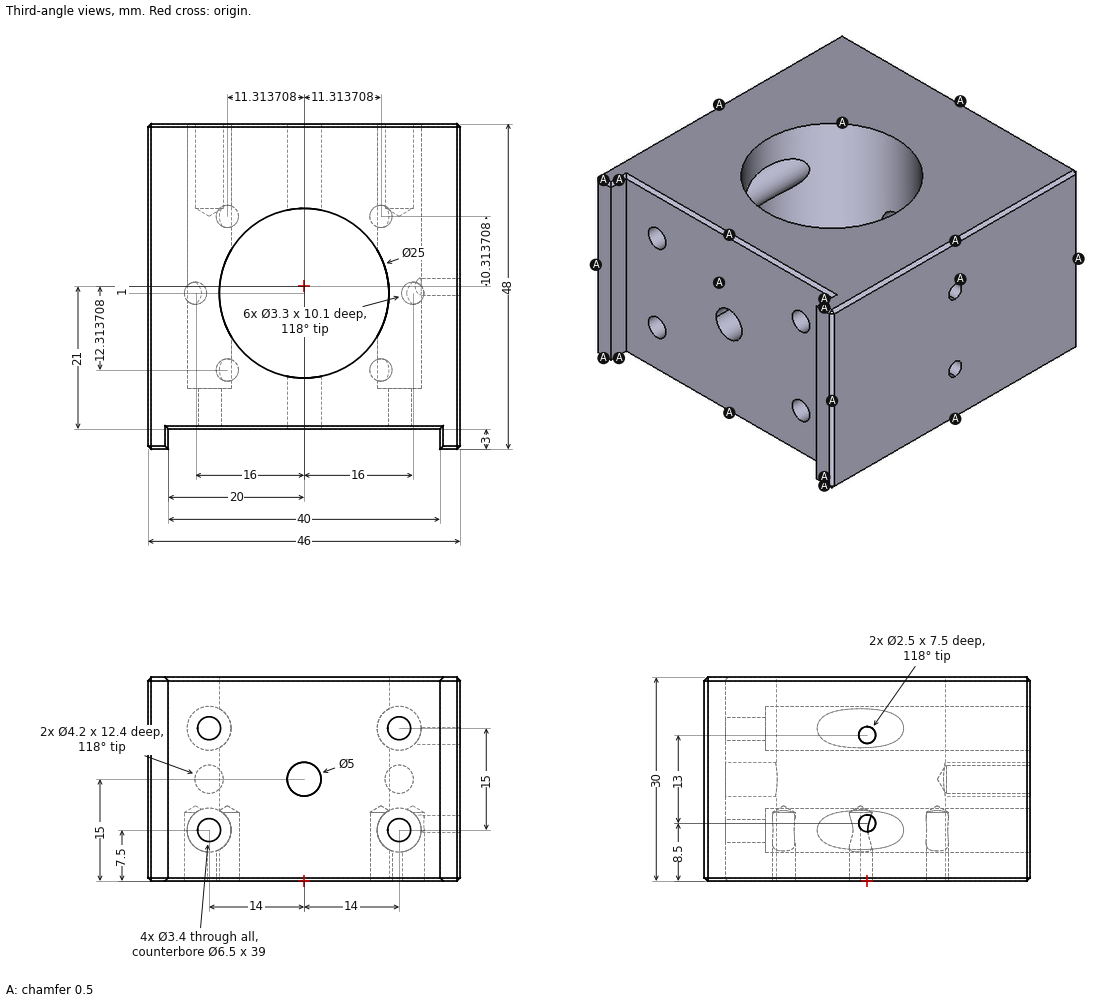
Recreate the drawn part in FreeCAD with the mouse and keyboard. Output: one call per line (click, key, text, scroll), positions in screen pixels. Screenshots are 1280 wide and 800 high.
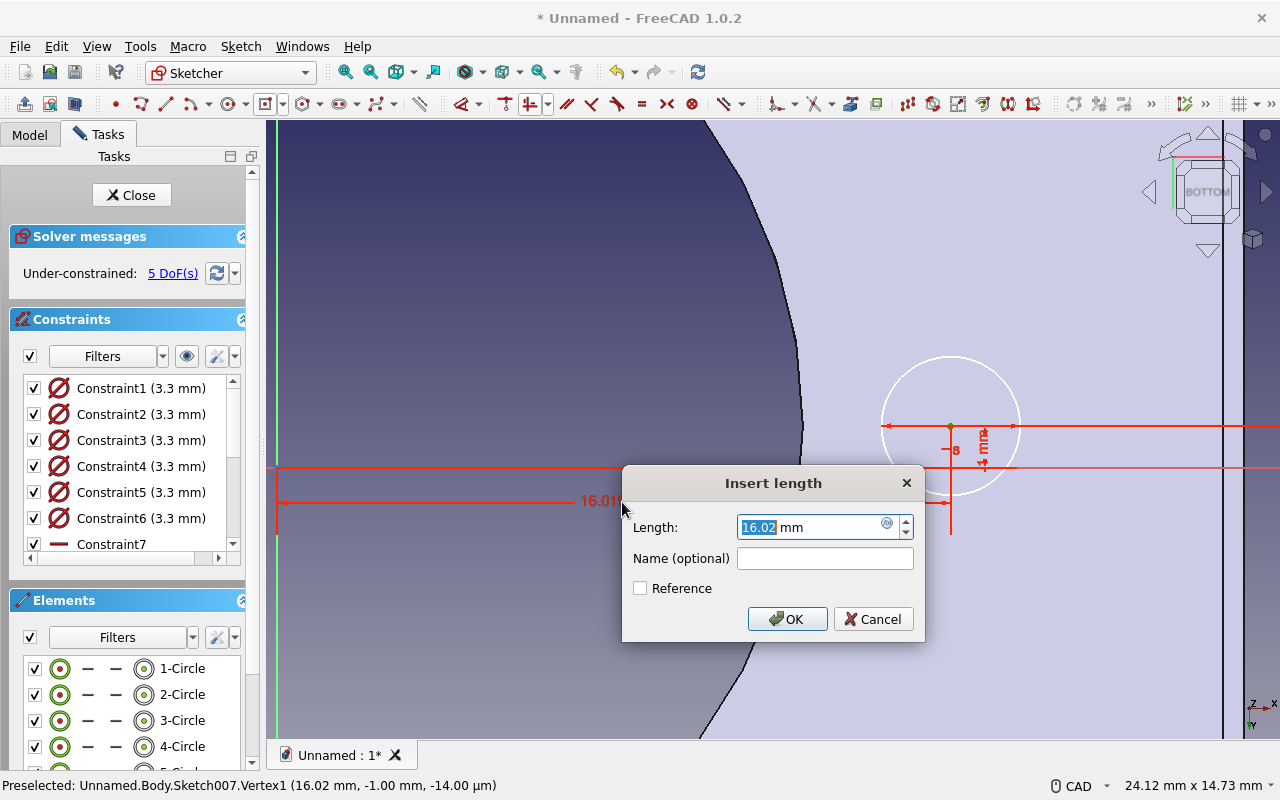
text(16)
key(Return)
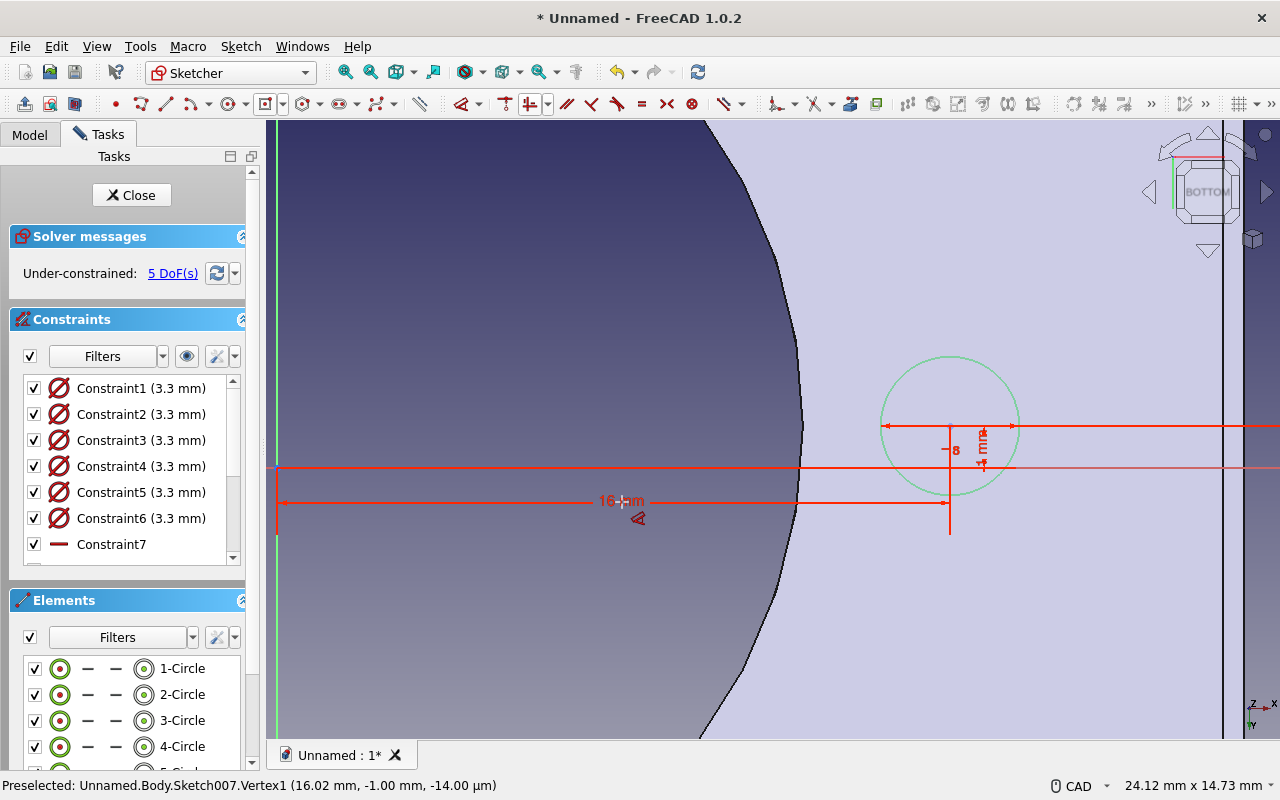
scroll(953, 432, down, 5)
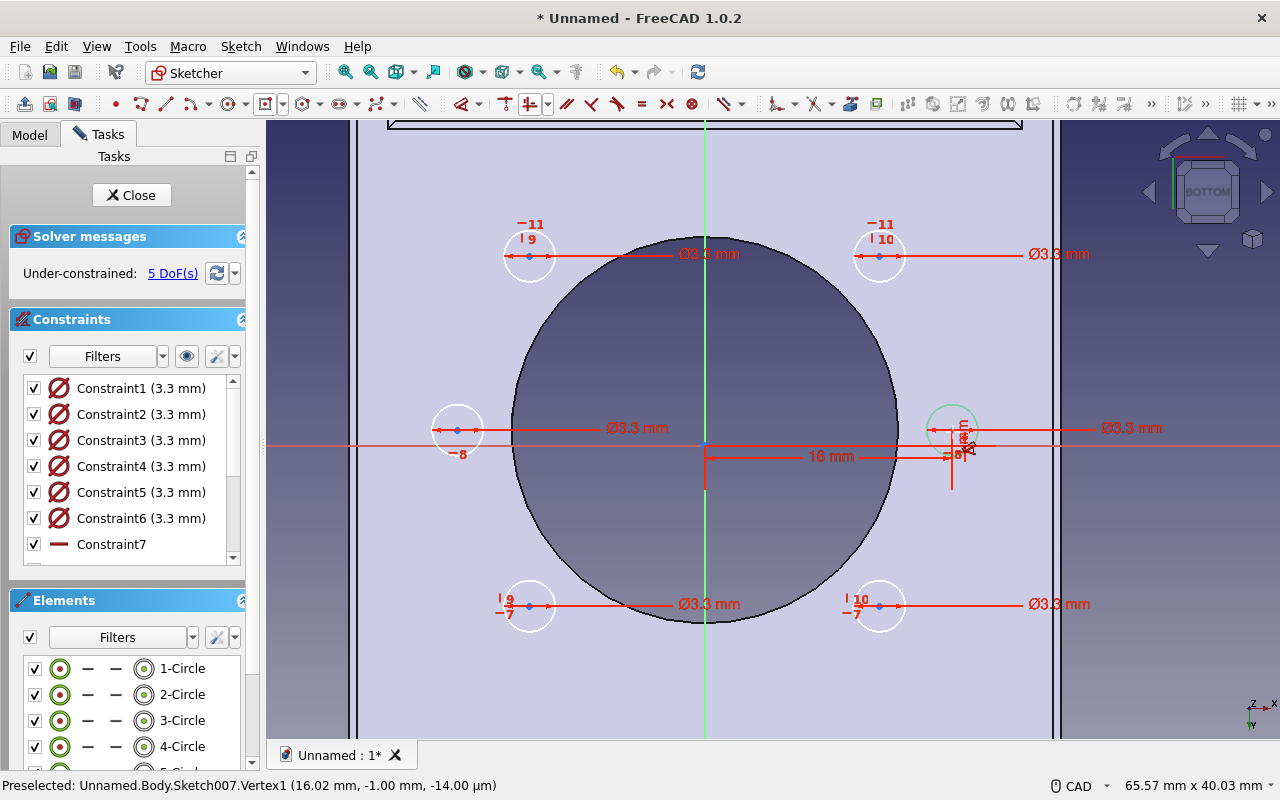
click(458, 430)
click(581, 480)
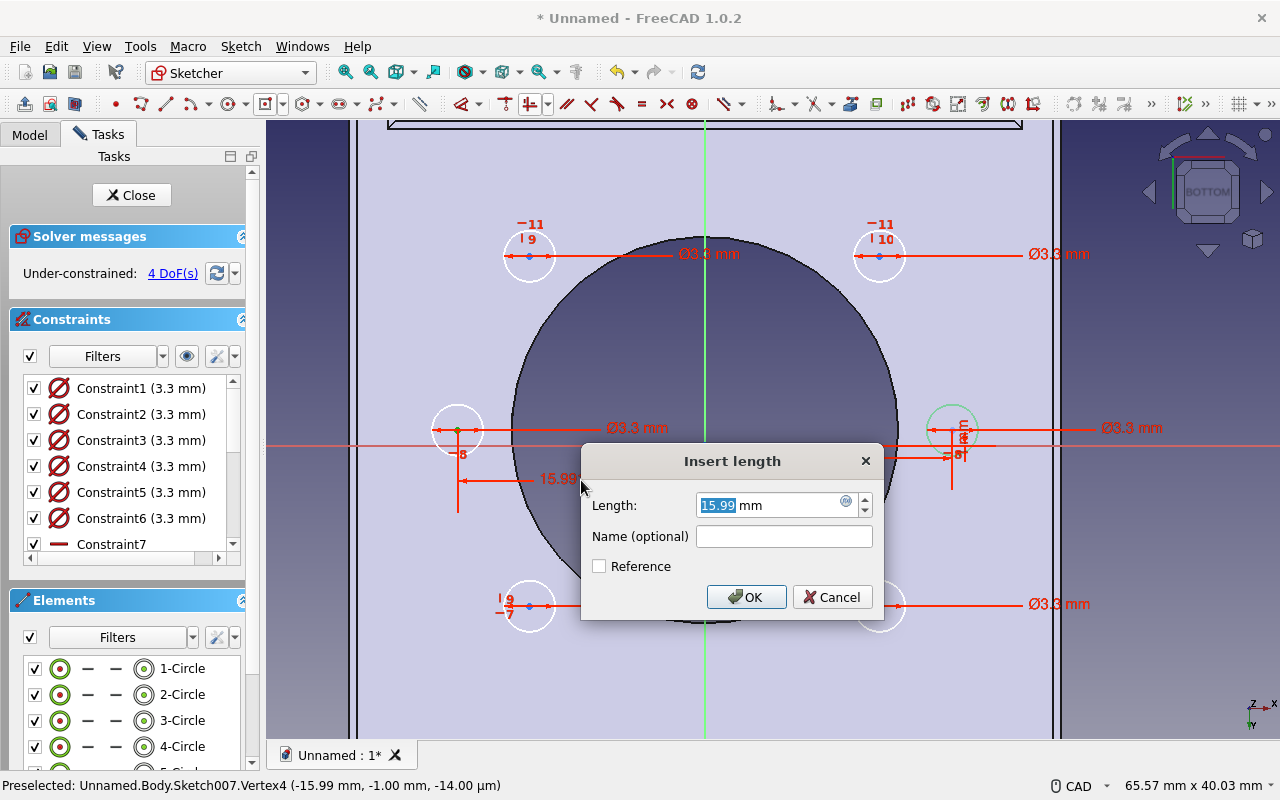
text(16)
key(Return)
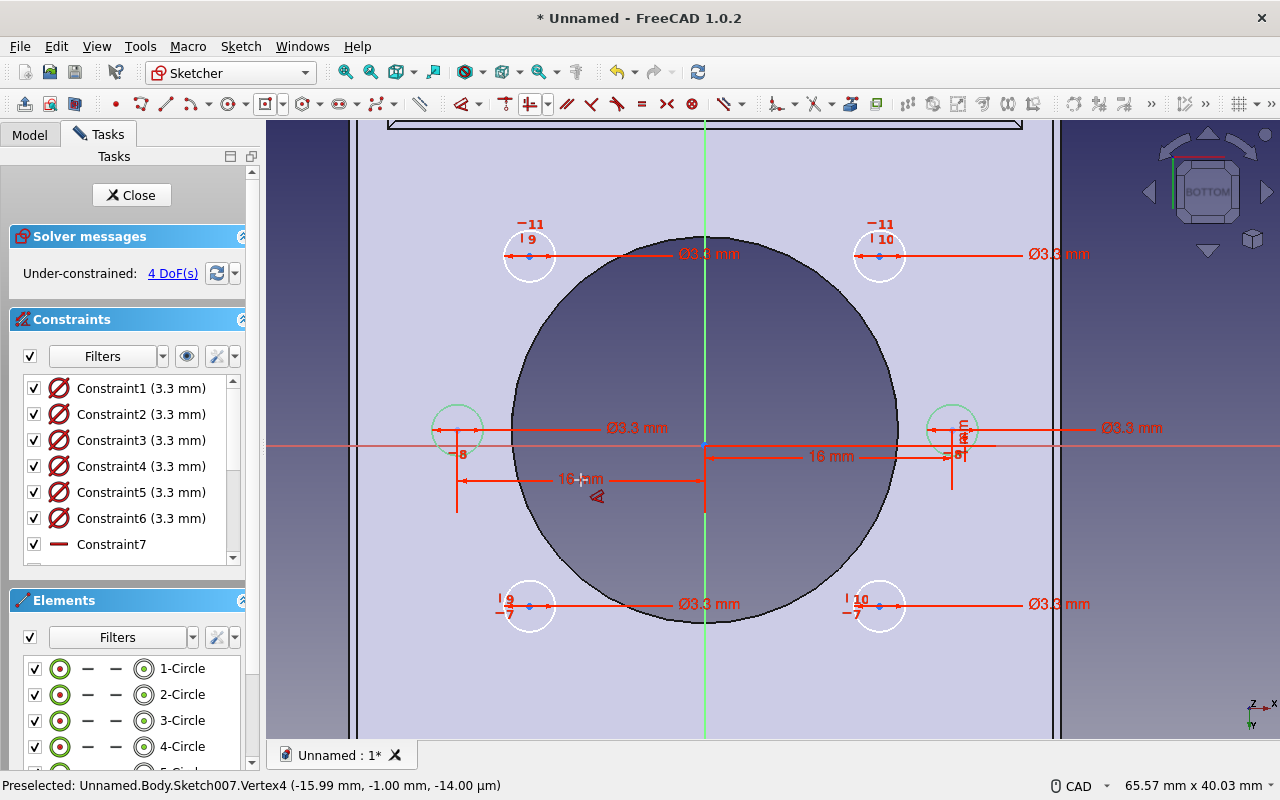
click(880, 606)
click(792, 640)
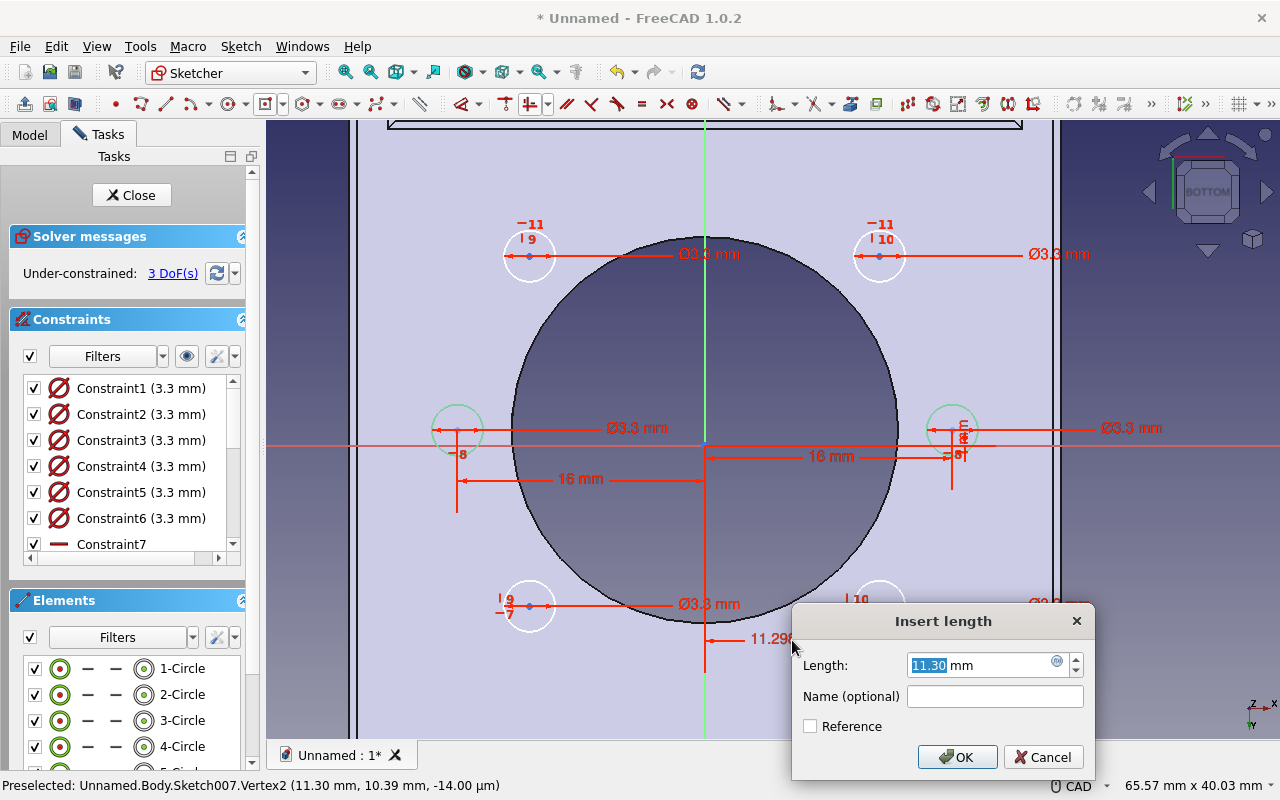
text(11.313708)
key(Return)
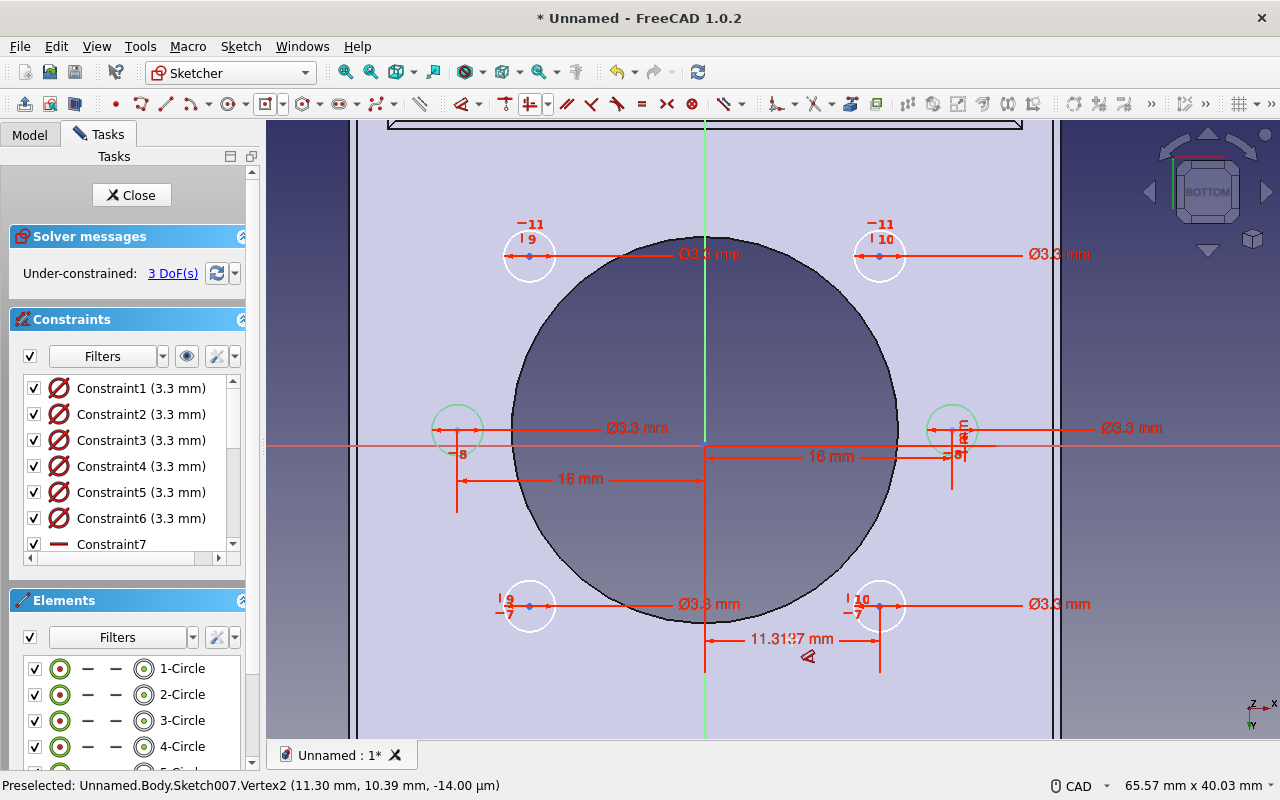
click(880, 606)
click(914, 526)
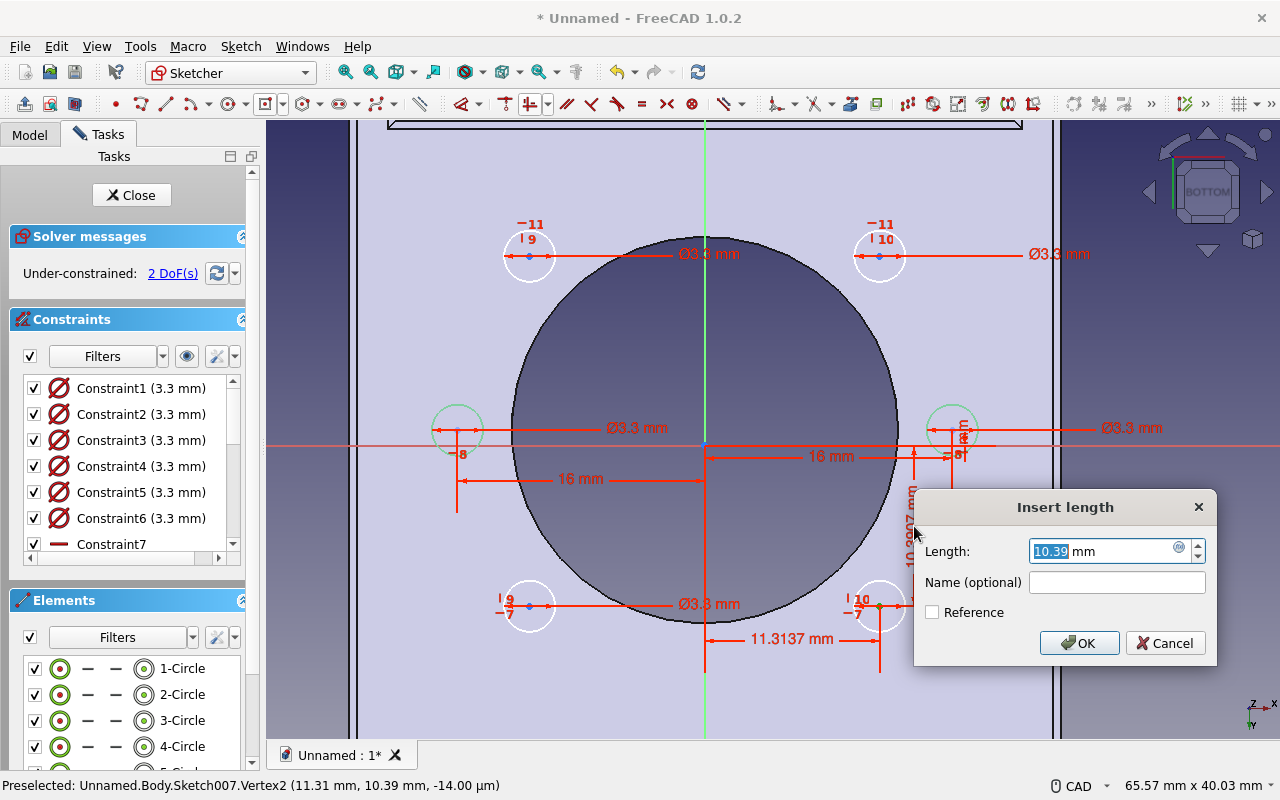
text(10.313708)
key(Return)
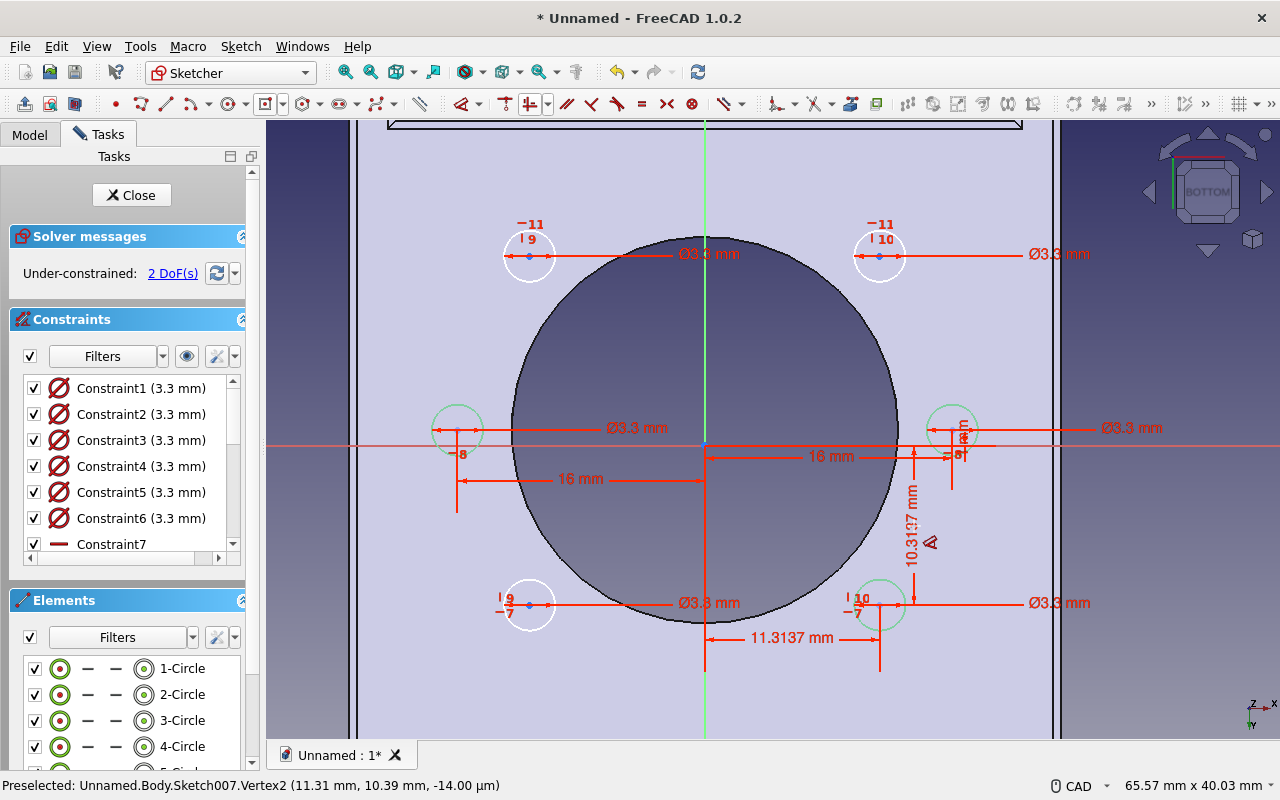
click(530, 605)
click(617, 639)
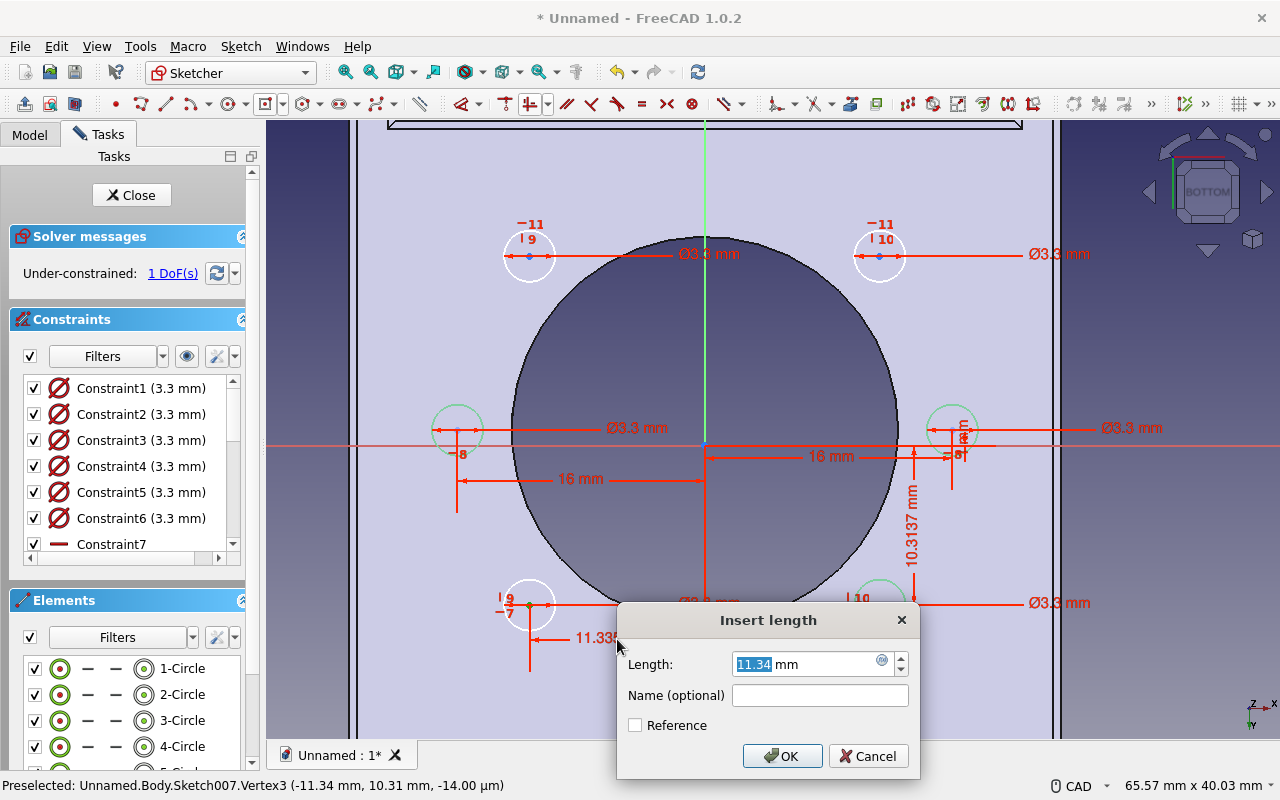
text(11.313708)
key(Return)